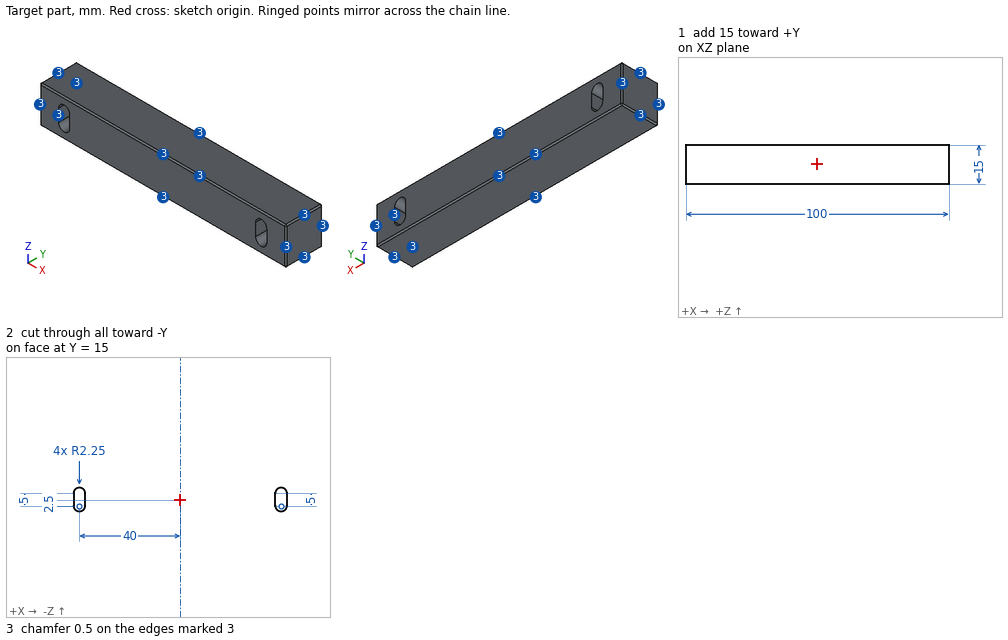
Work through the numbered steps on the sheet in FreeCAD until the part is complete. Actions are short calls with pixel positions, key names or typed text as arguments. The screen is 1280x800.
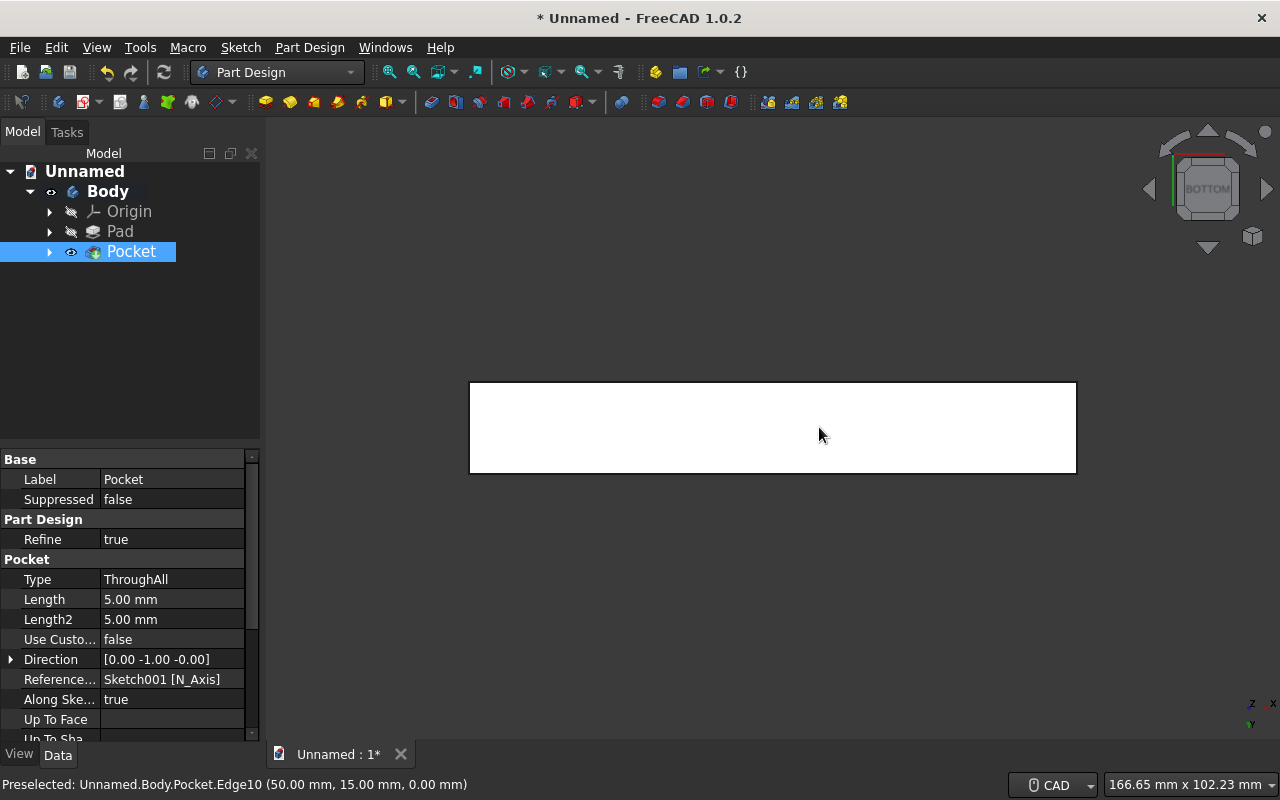
click(947, 427, ctrl)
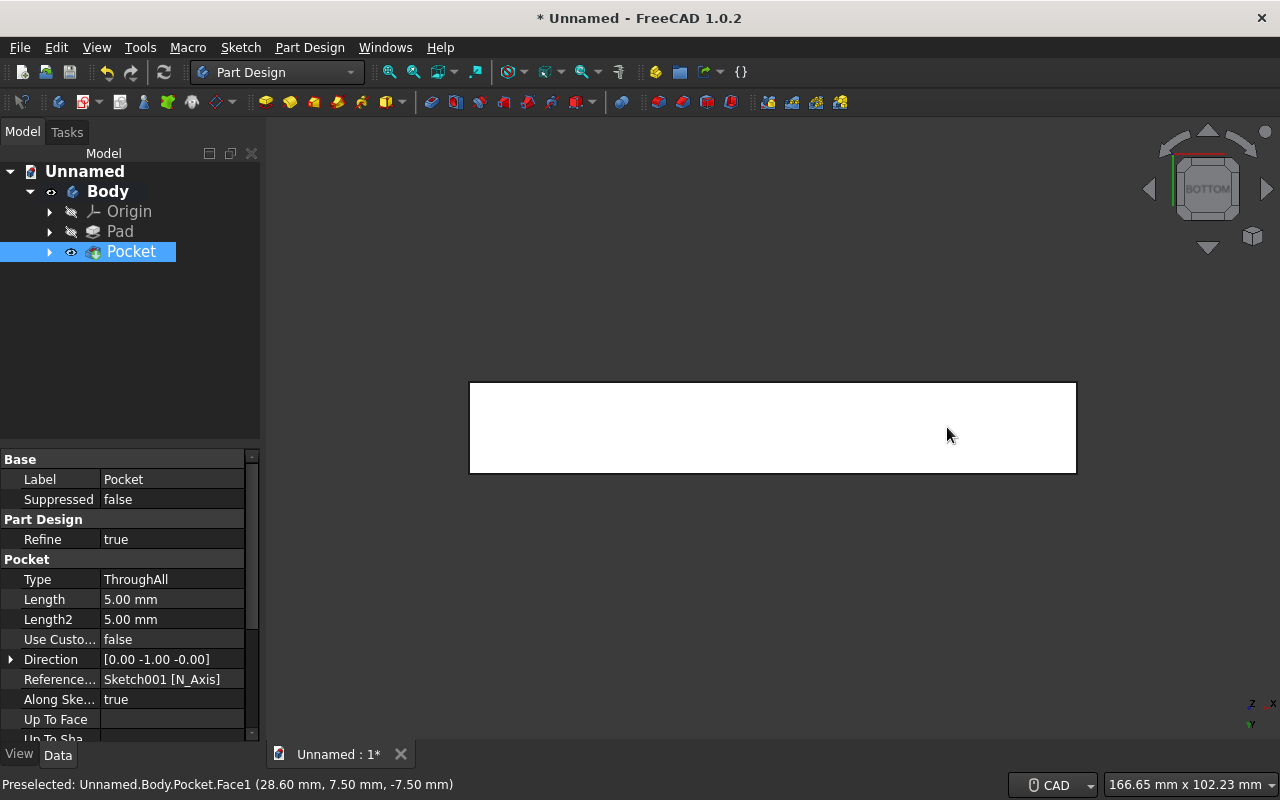
key(4)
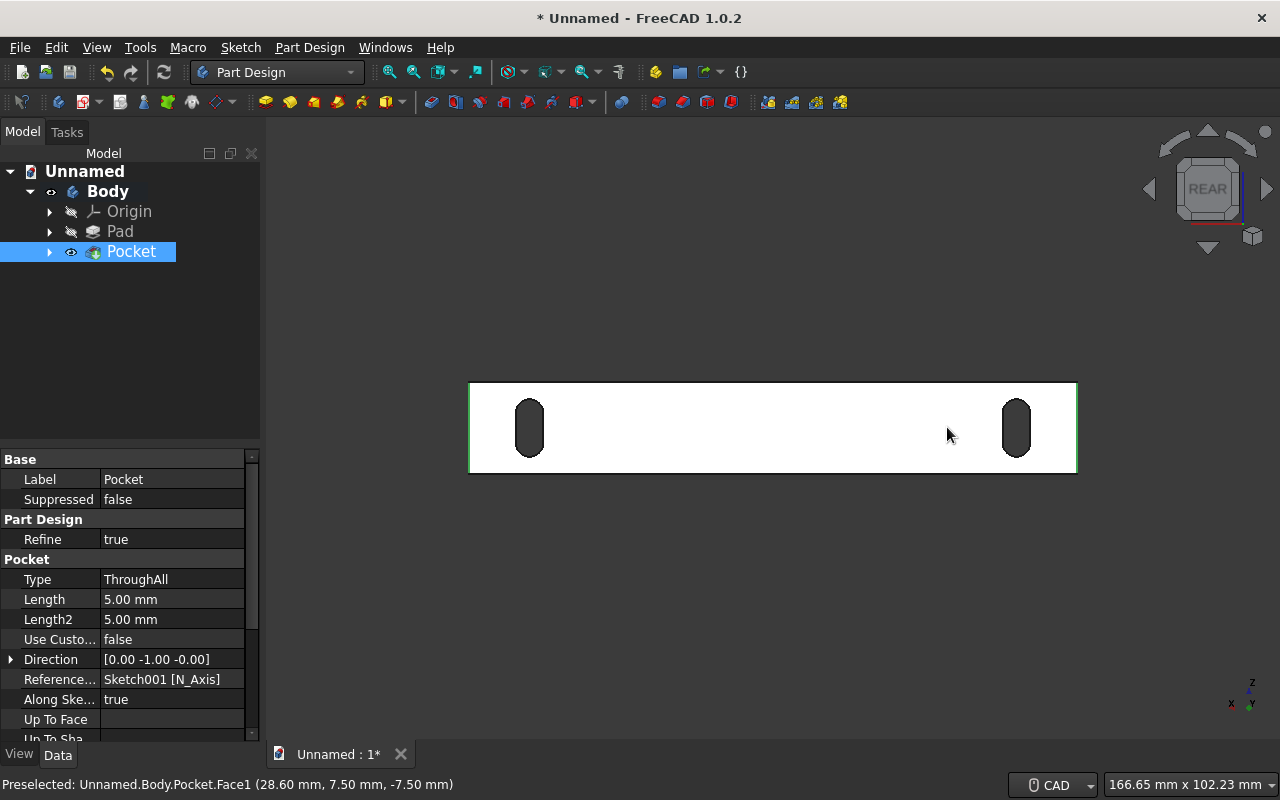
key(6)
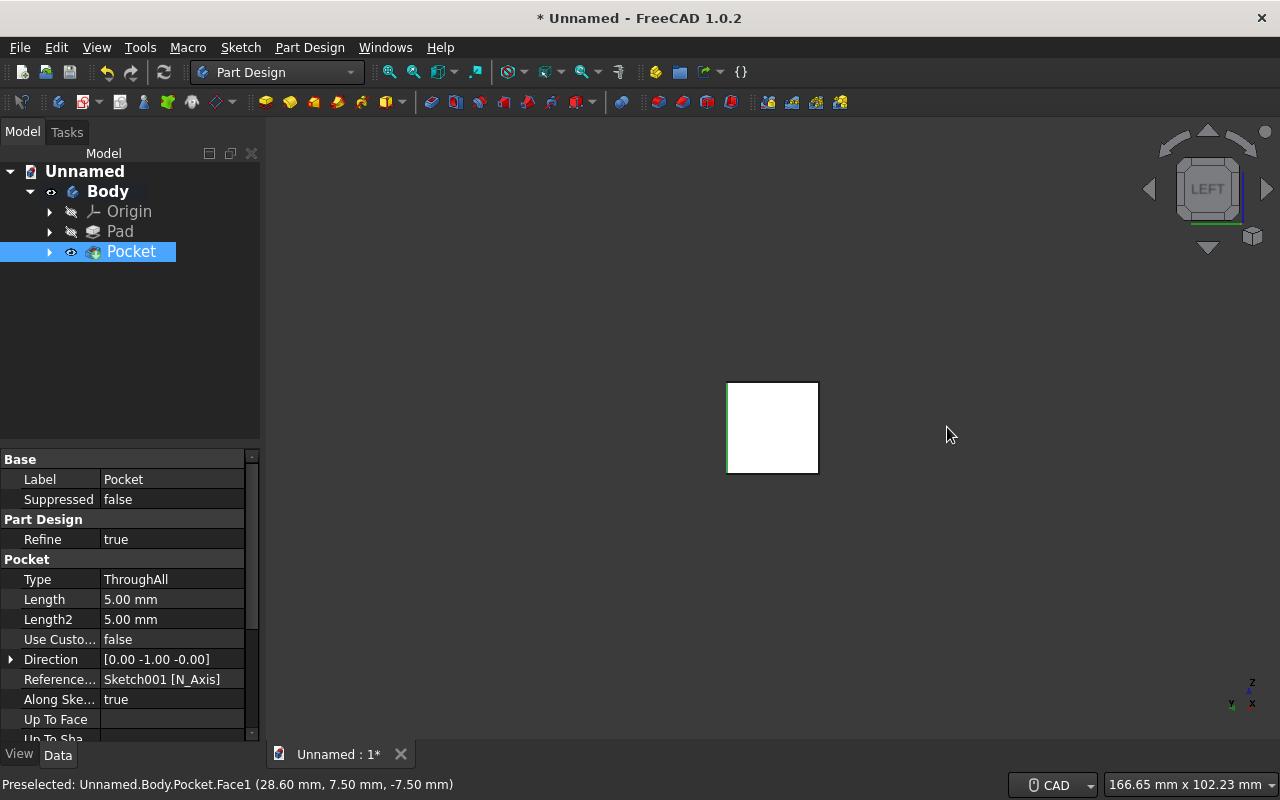
click(390, 72)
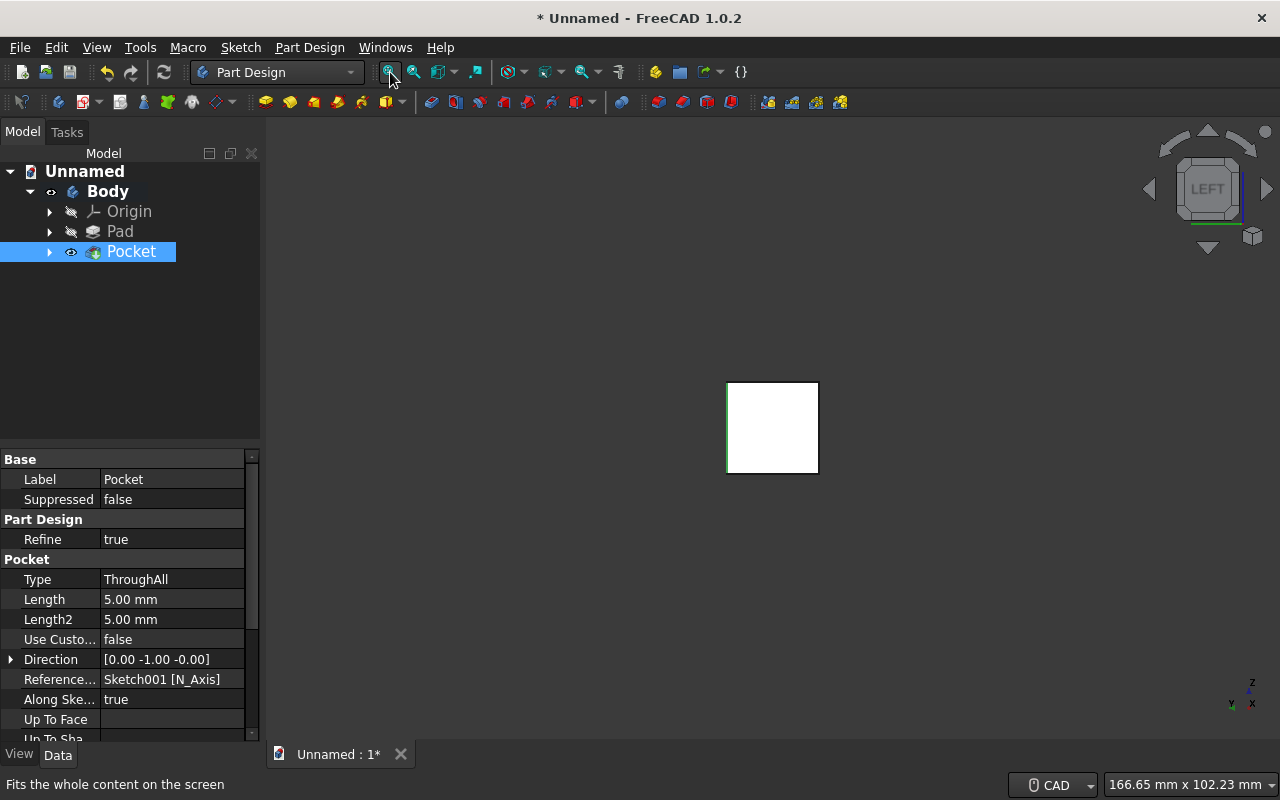
click(819, 427, ctrl)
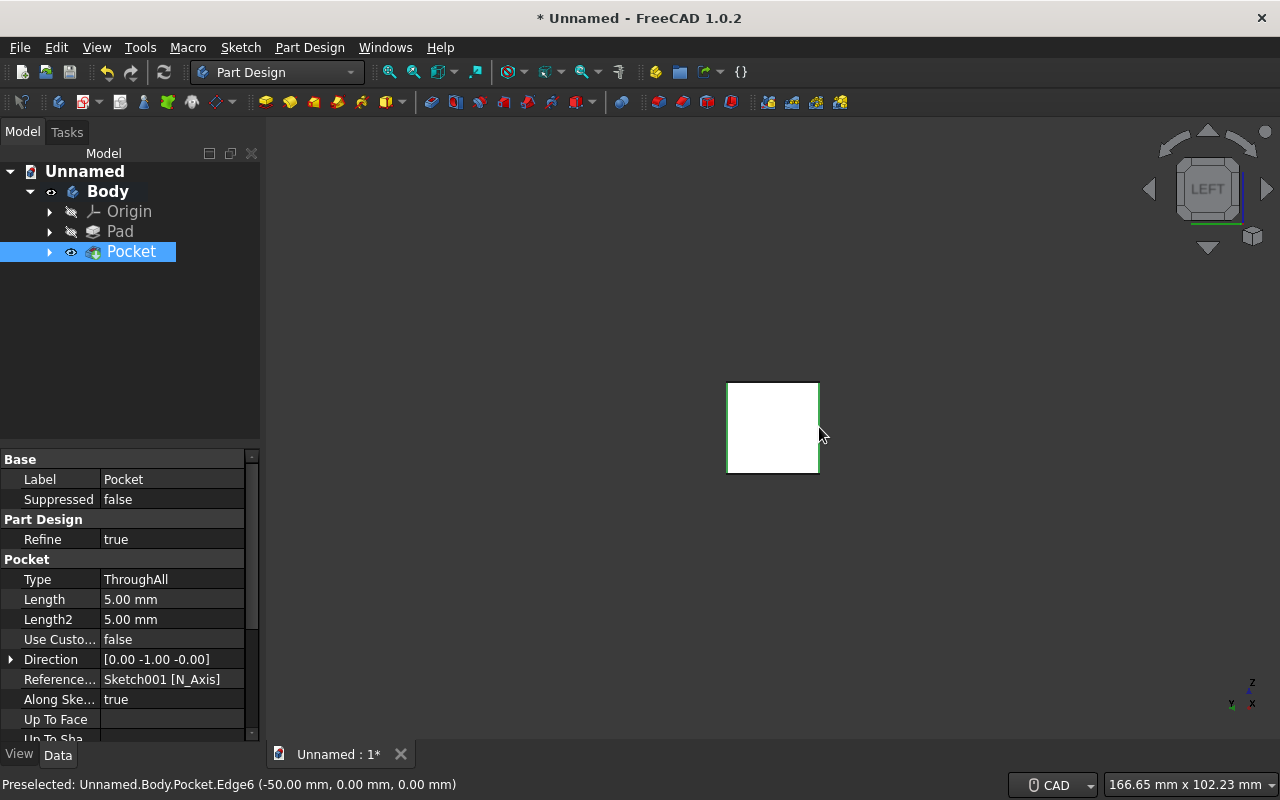
click(684, 102)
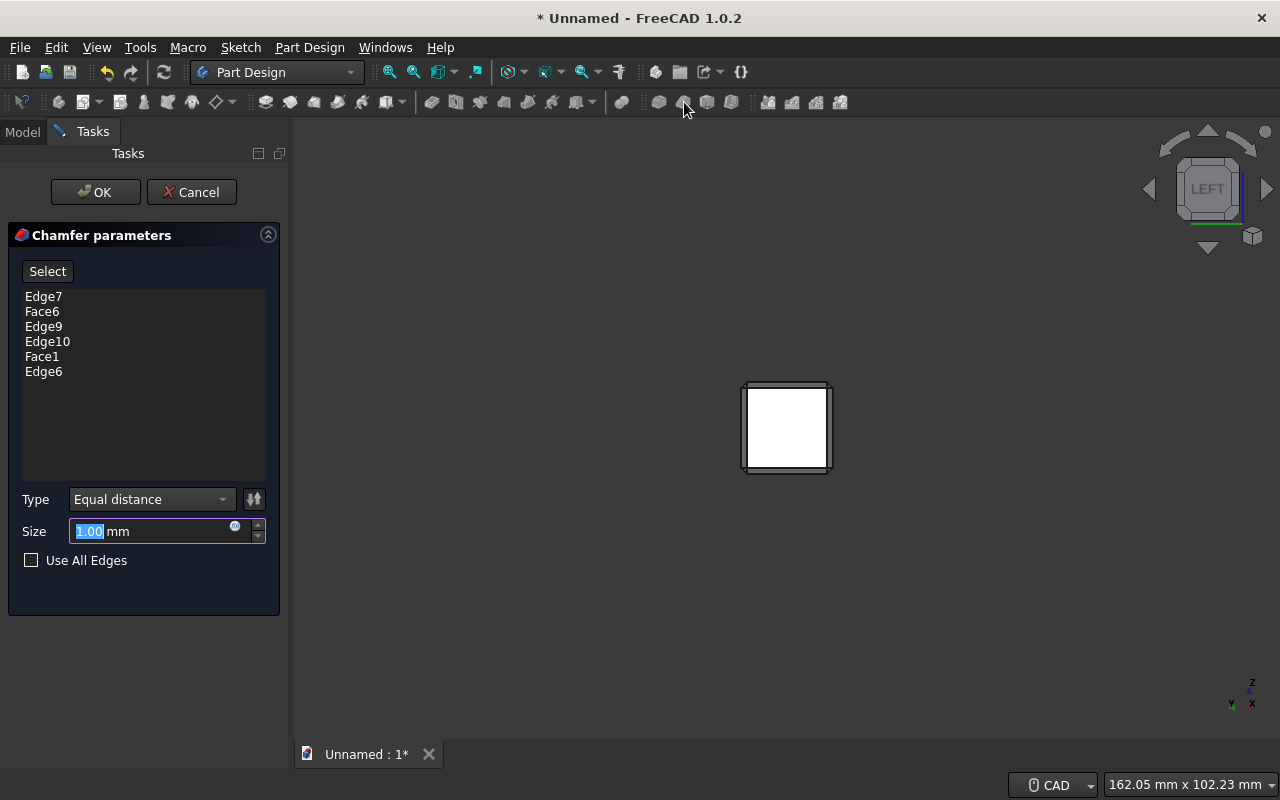
text(0.5)
key(Tab)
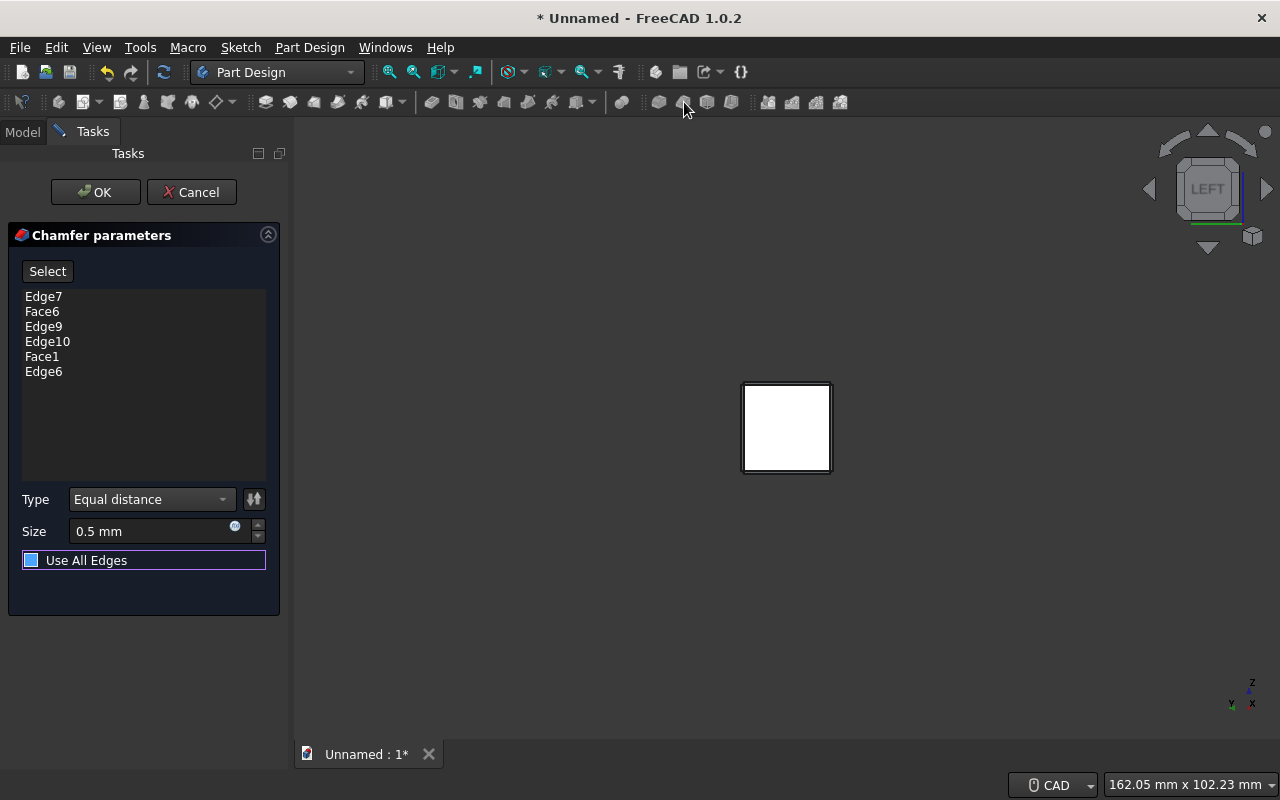
click(96, 192)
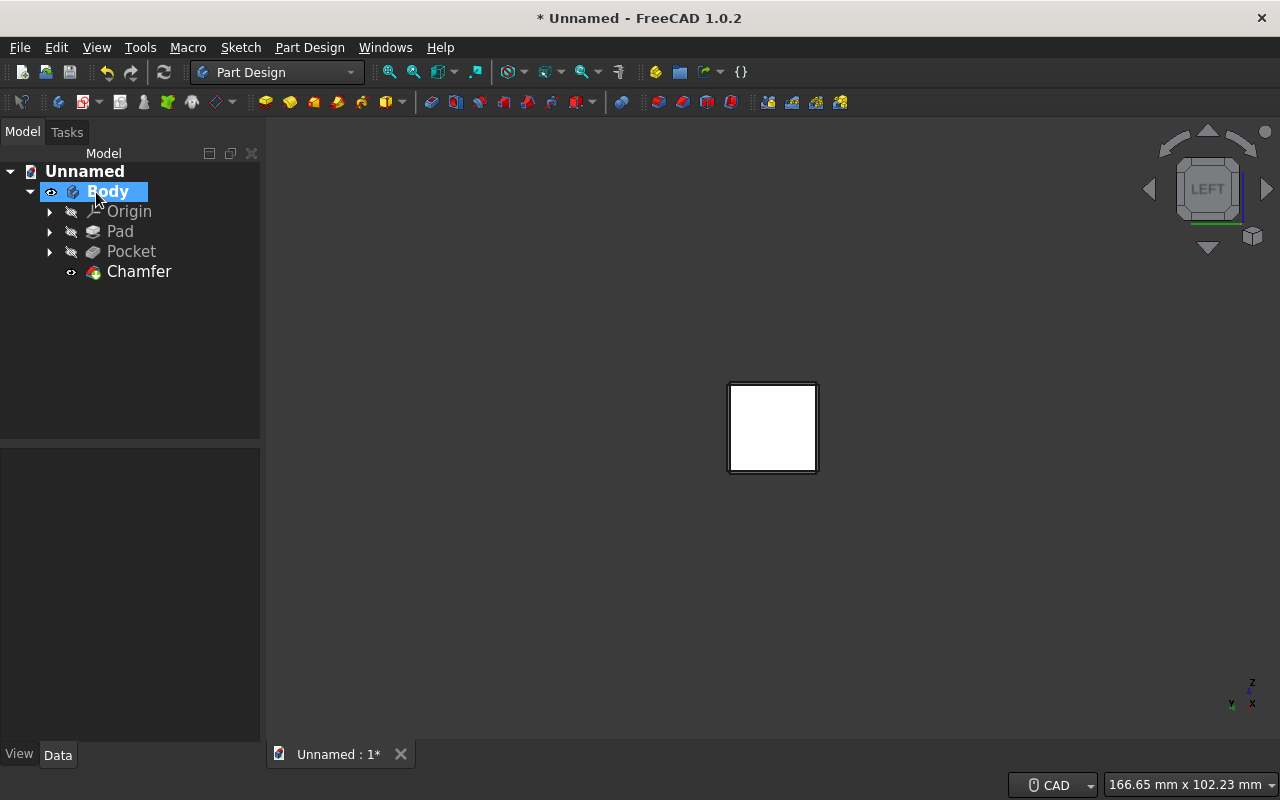
key(0)